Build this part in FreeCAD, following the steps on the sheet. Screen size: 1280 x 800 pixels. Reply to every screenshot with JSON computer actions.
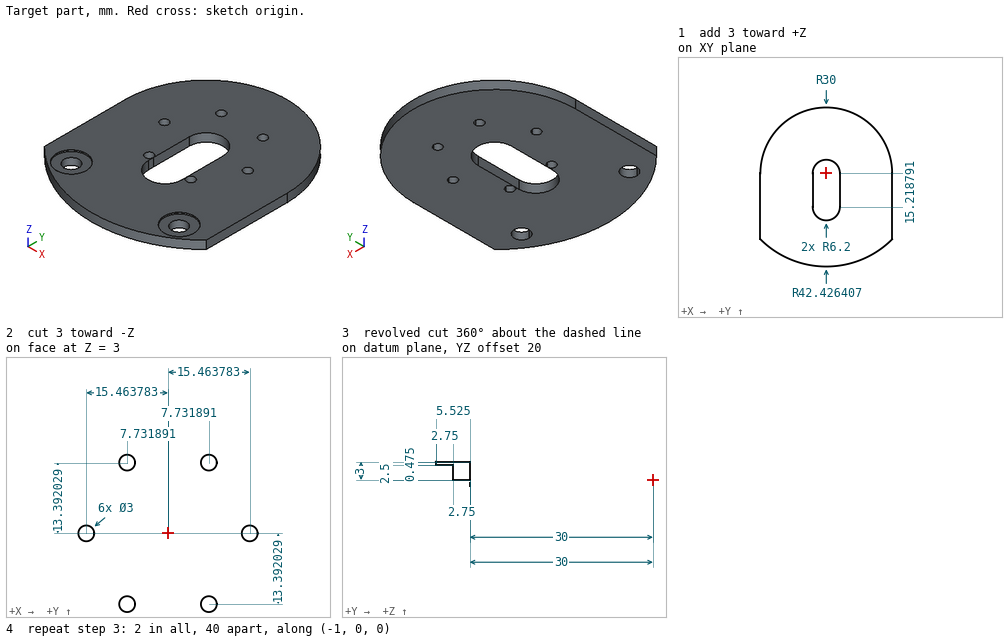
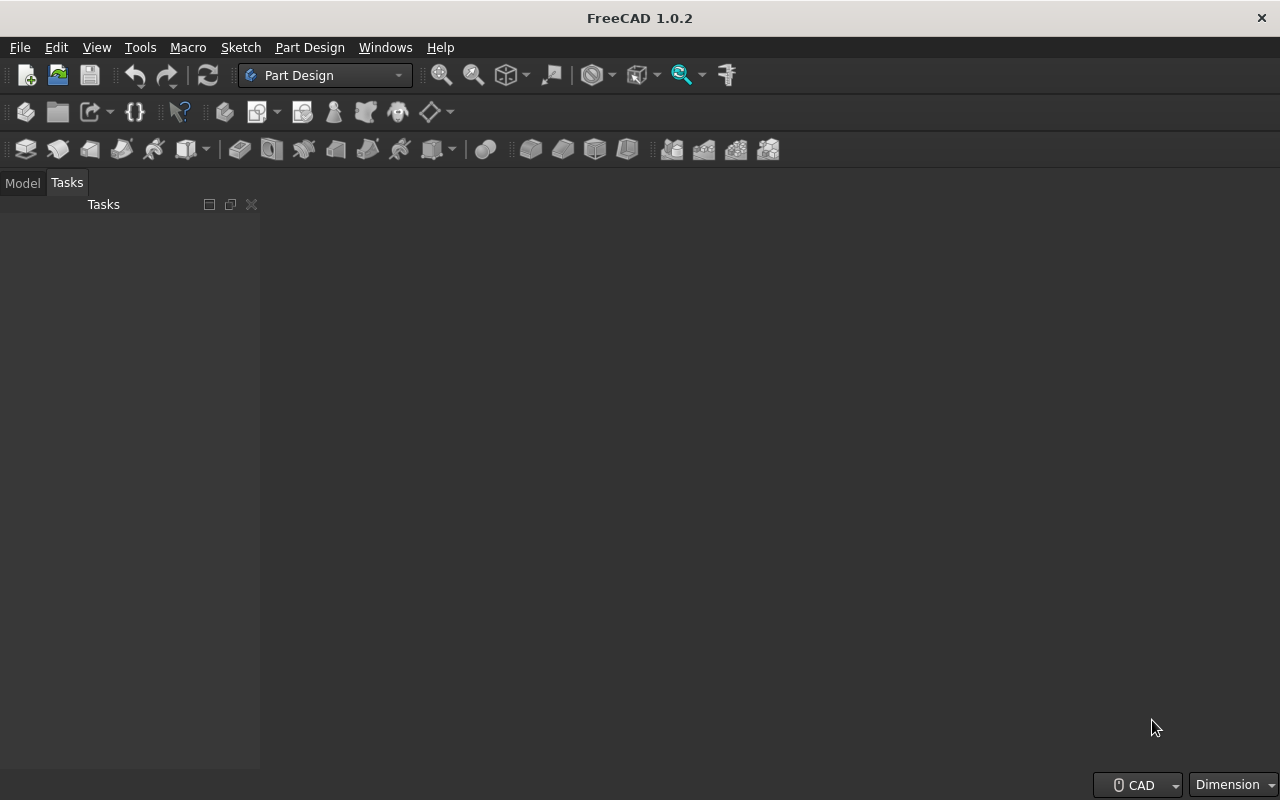
{"action": "key", "text": "ctrl+n"}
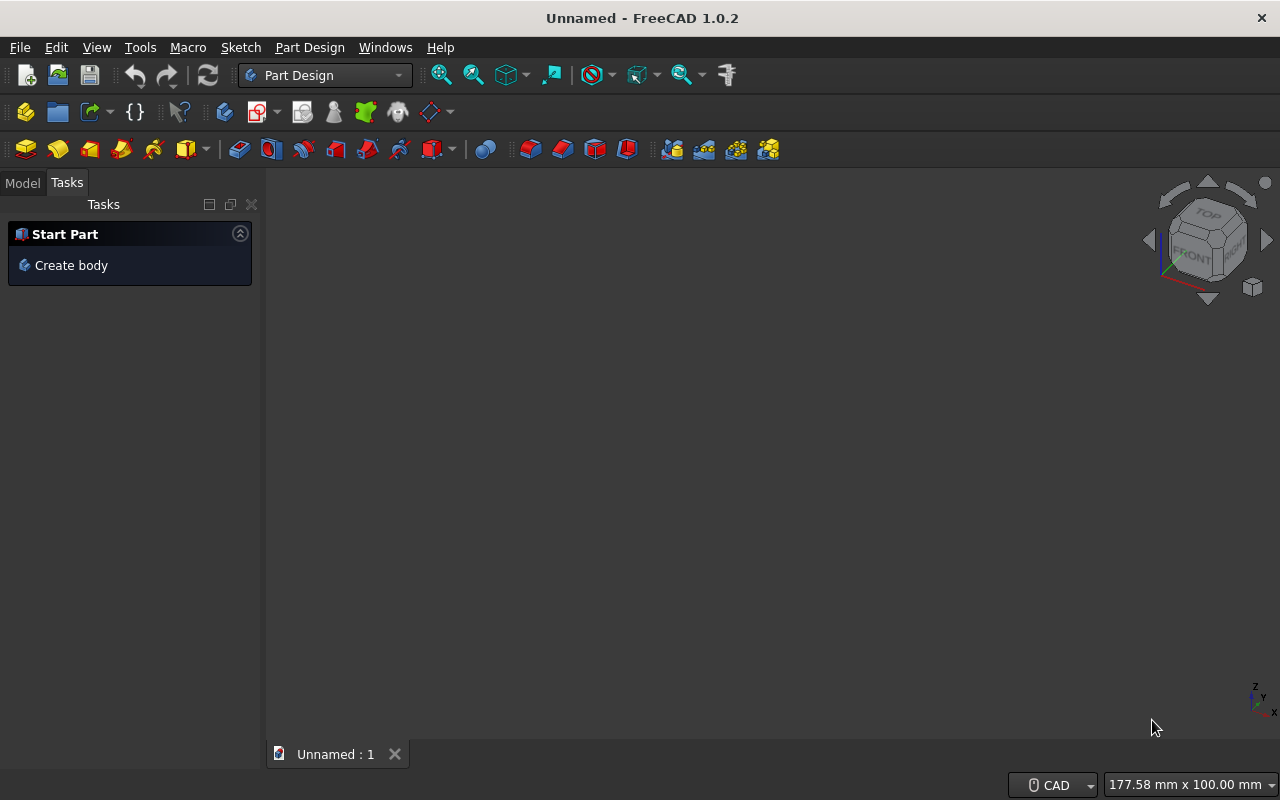
{"action": "left_click", "coordinate": [258, 112]}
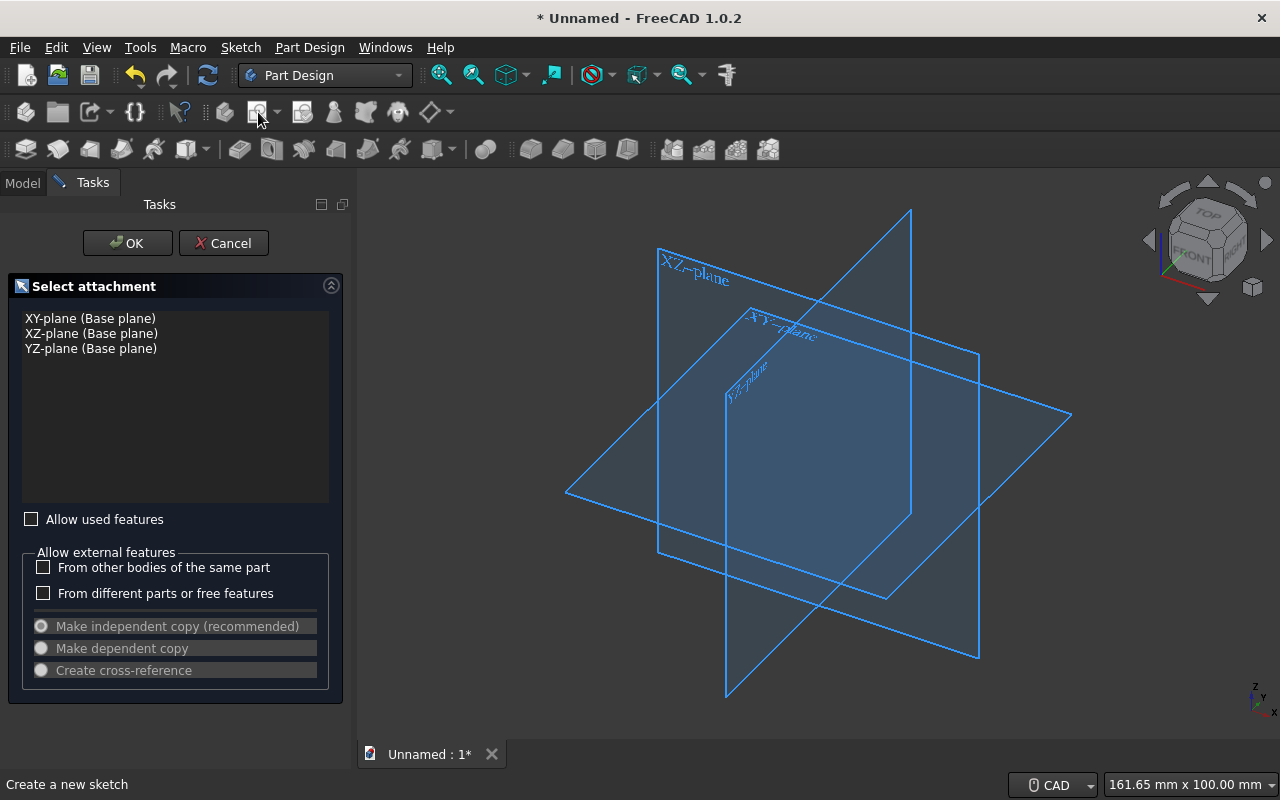
{"action": "left_click", "coordinate": [82, 318]}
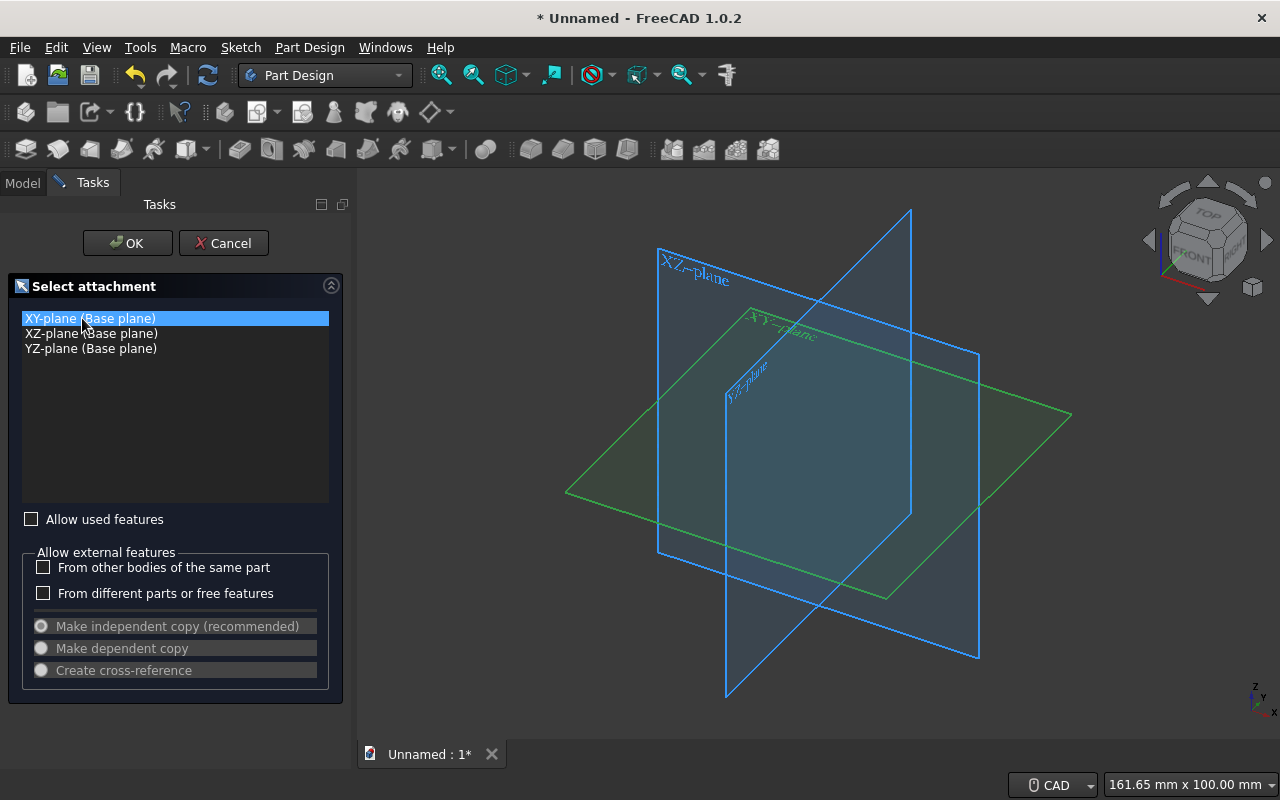
{"action": "left_click", "coordinate": [128, 243]}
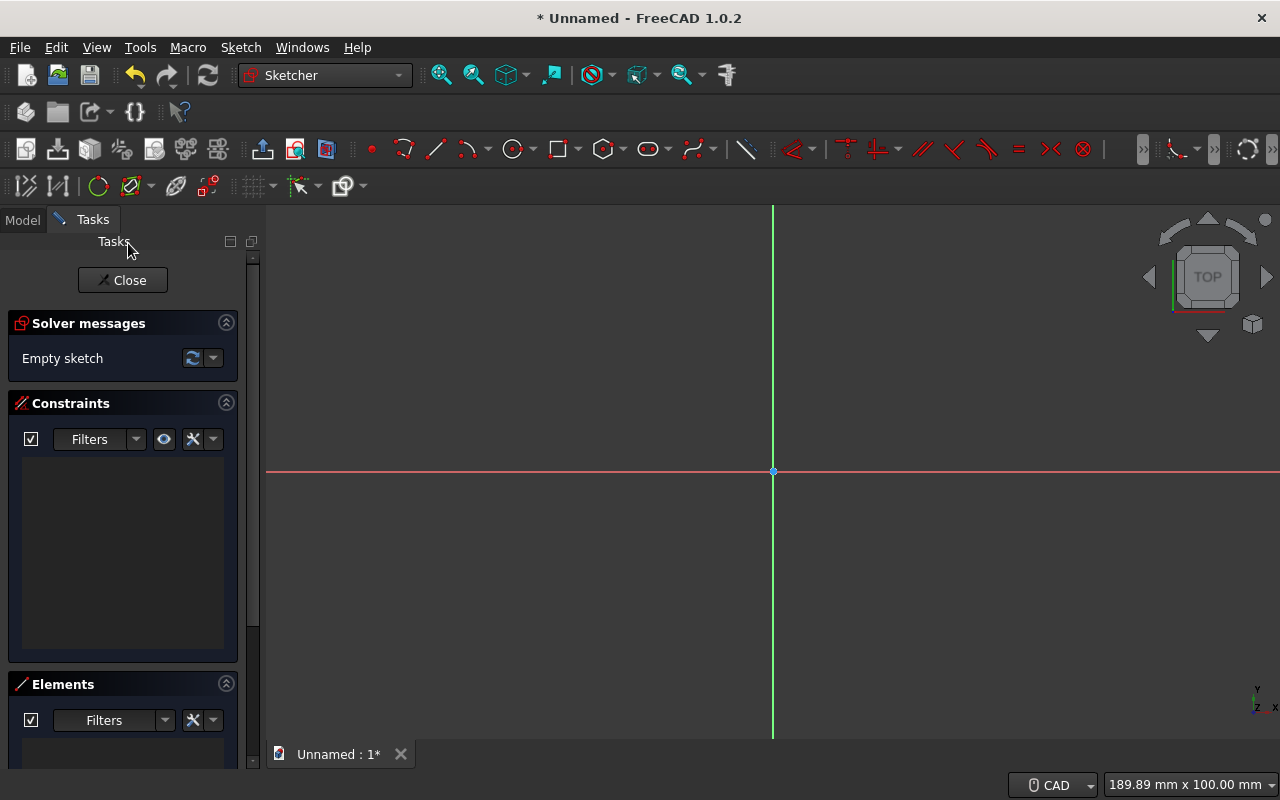
{"action": "scroll", "coordinate": [395, 322], "scroll_direction": "down", "scroll_amount": 1}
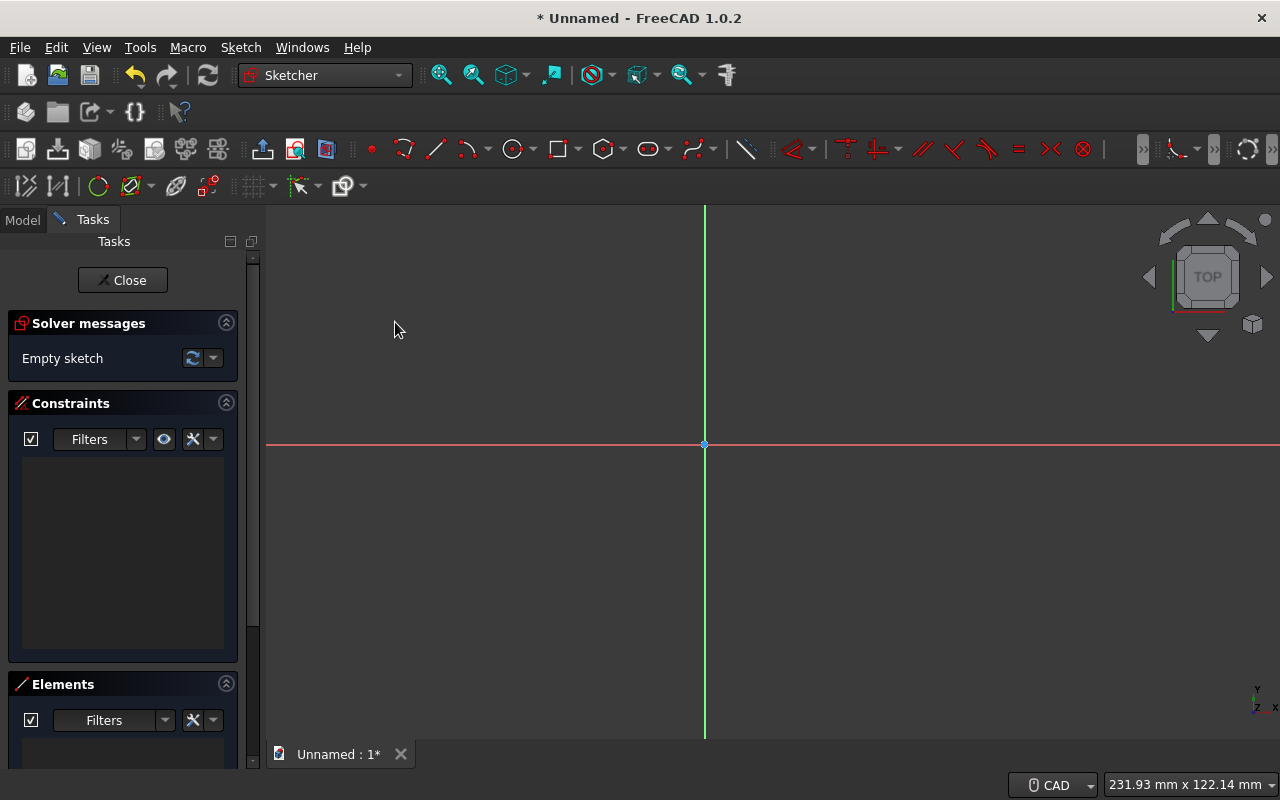
{"action": "key", "text": "g l"}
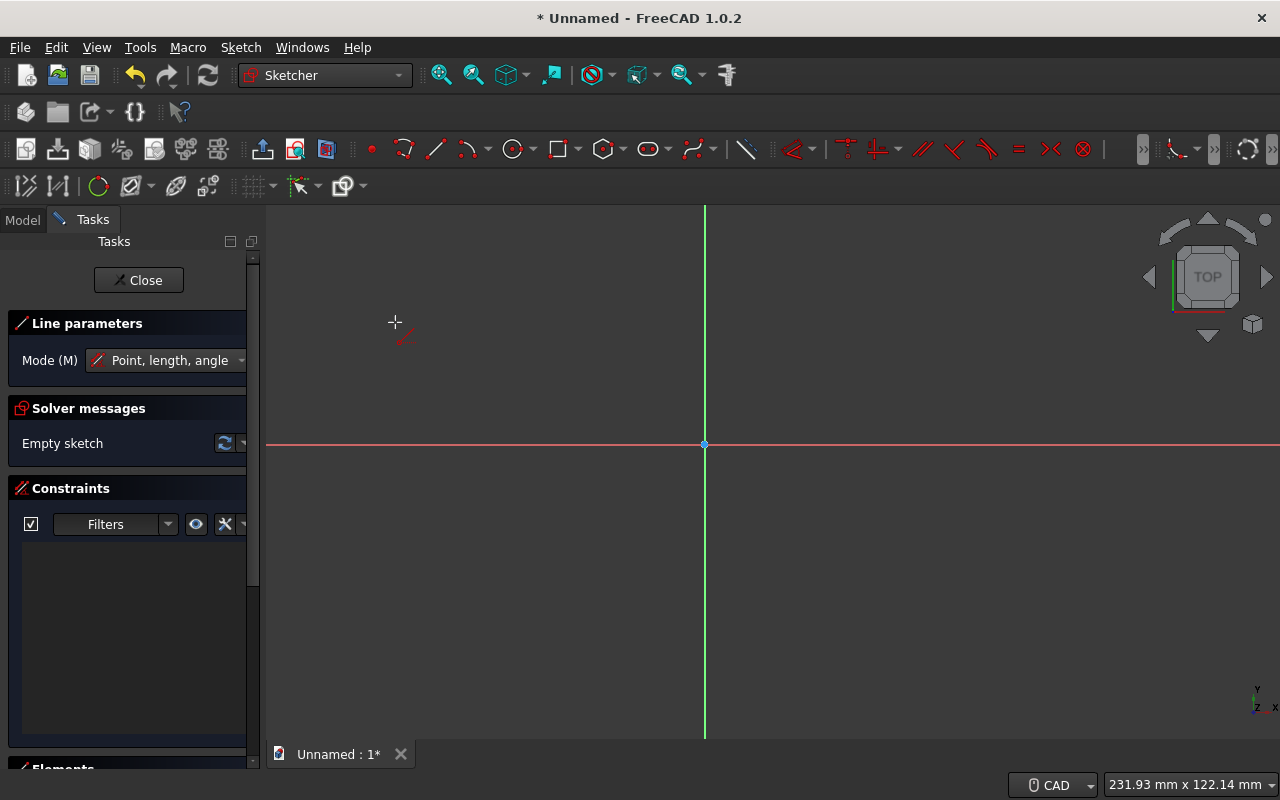
{"action": "left_click", "coordinate": [836, 576]}
{"action": "left_click", "coordinate": [836, 445]}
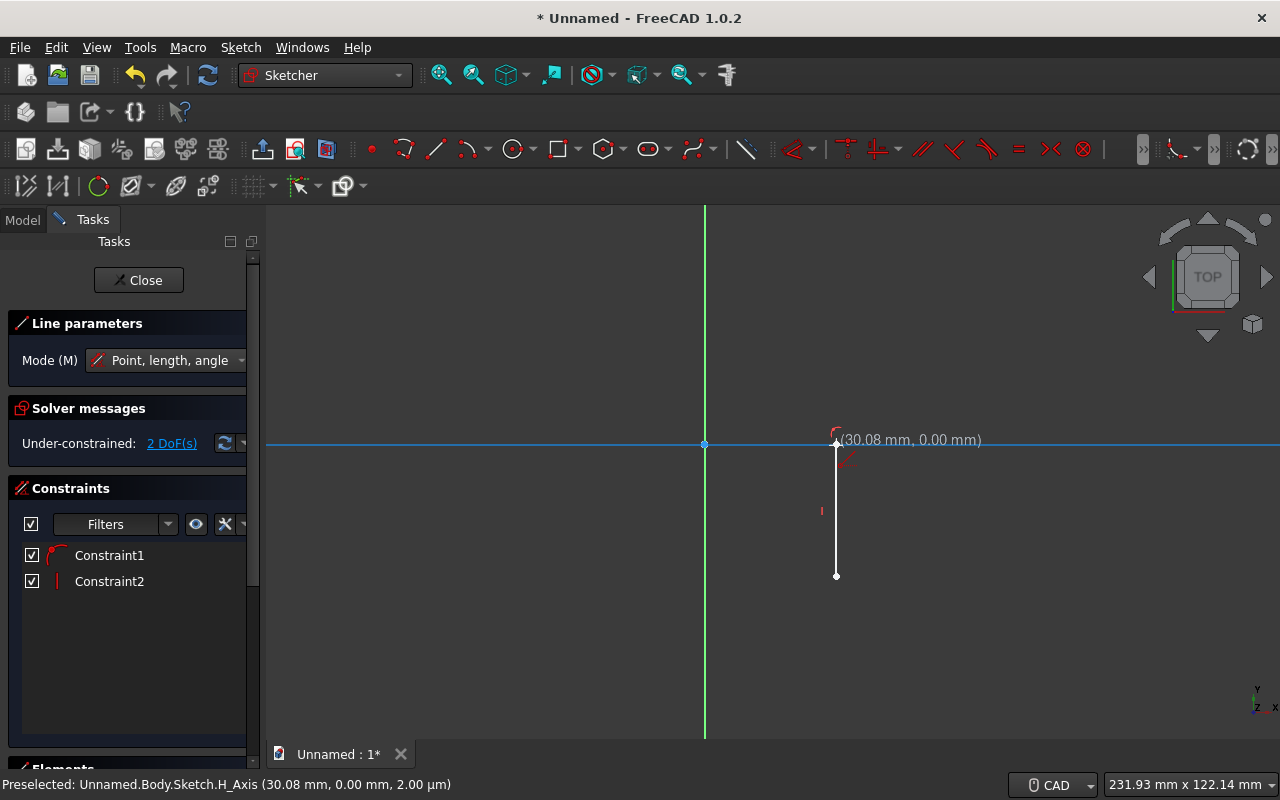
{"action": "left_click", "coordinate": [573, 445]}
{"action": "left_click", "coordinate": [573, 576]}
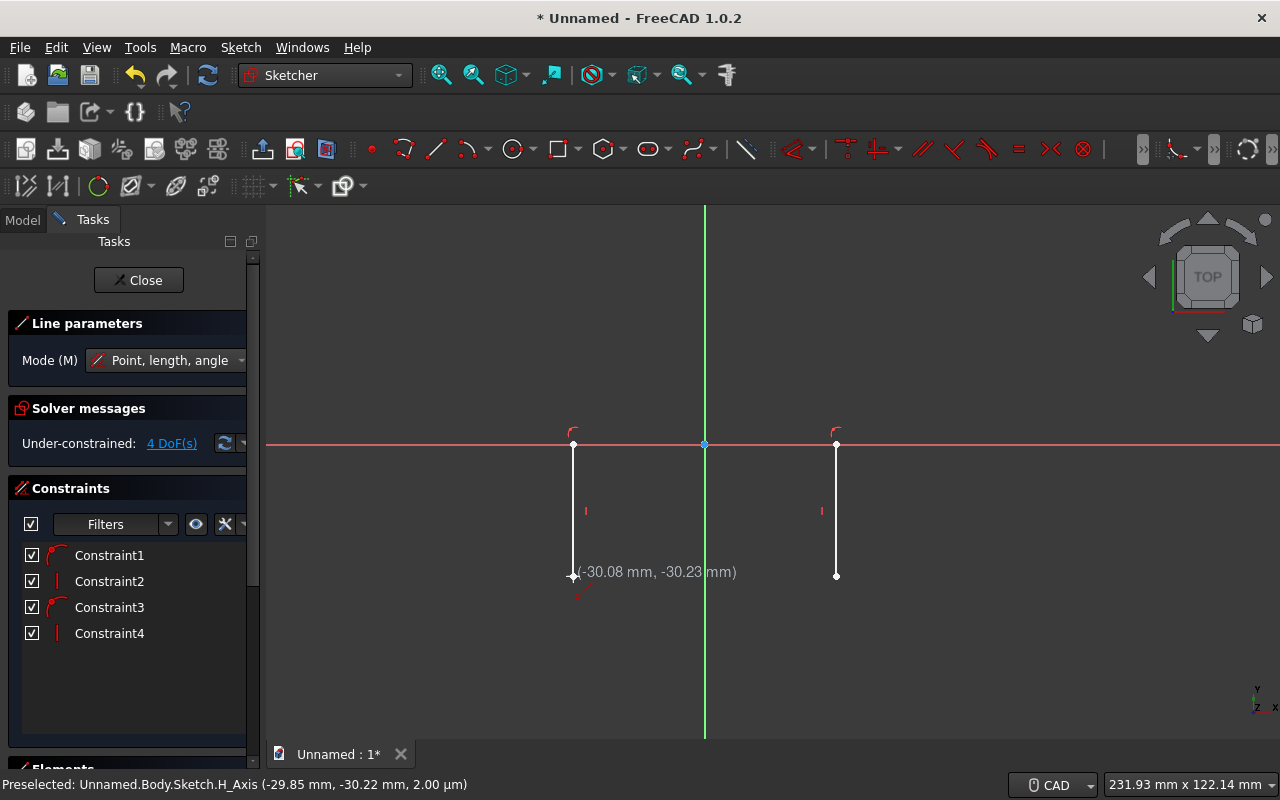
{"action": "key", "text": "g 3 a"}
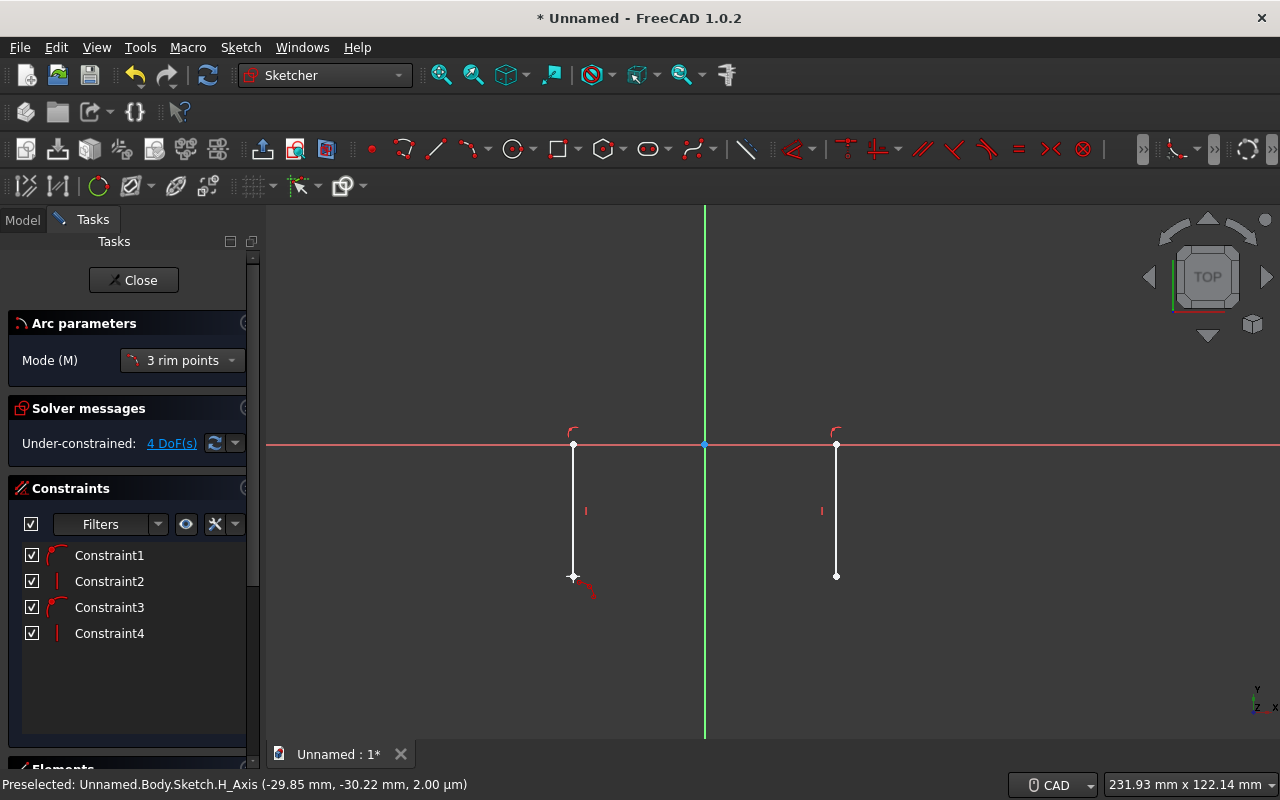
{"action": "left_click", "coordinate": [836, 445]}
{"action": "left_click", "coordinate": [573, 445]}
{"action": "left_click", "coordinate": [745, 320]}